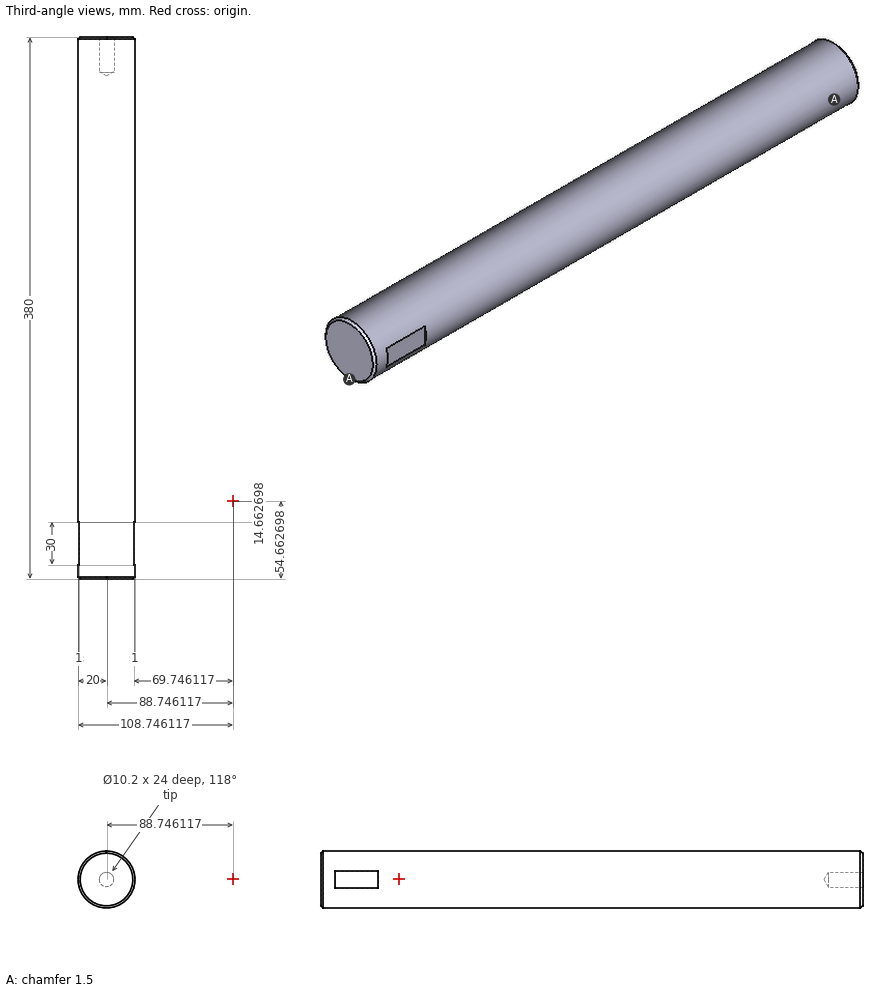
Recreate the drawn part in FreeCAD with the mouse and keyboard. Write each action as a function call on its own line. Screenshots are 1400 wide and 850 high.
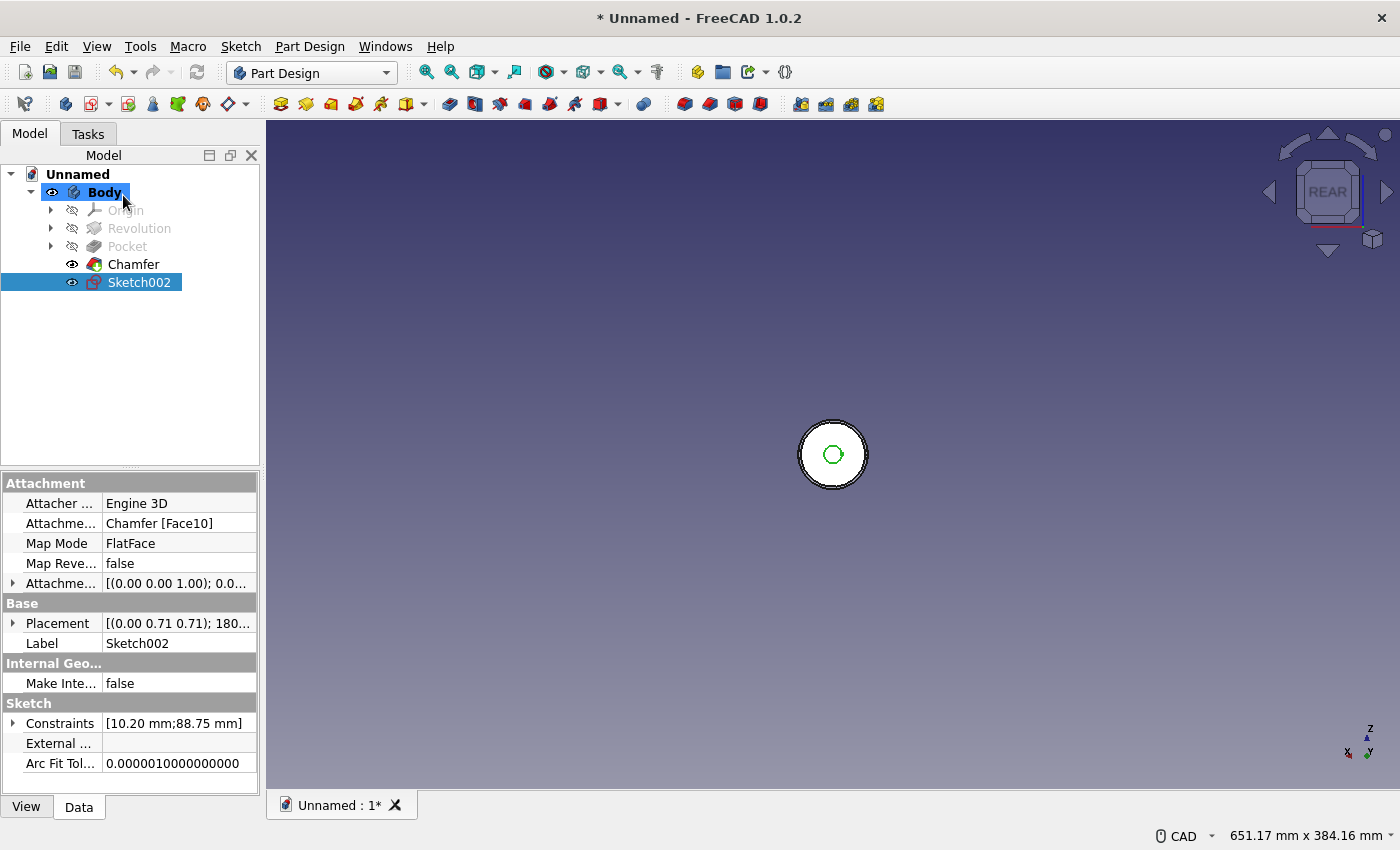
click(475, 104)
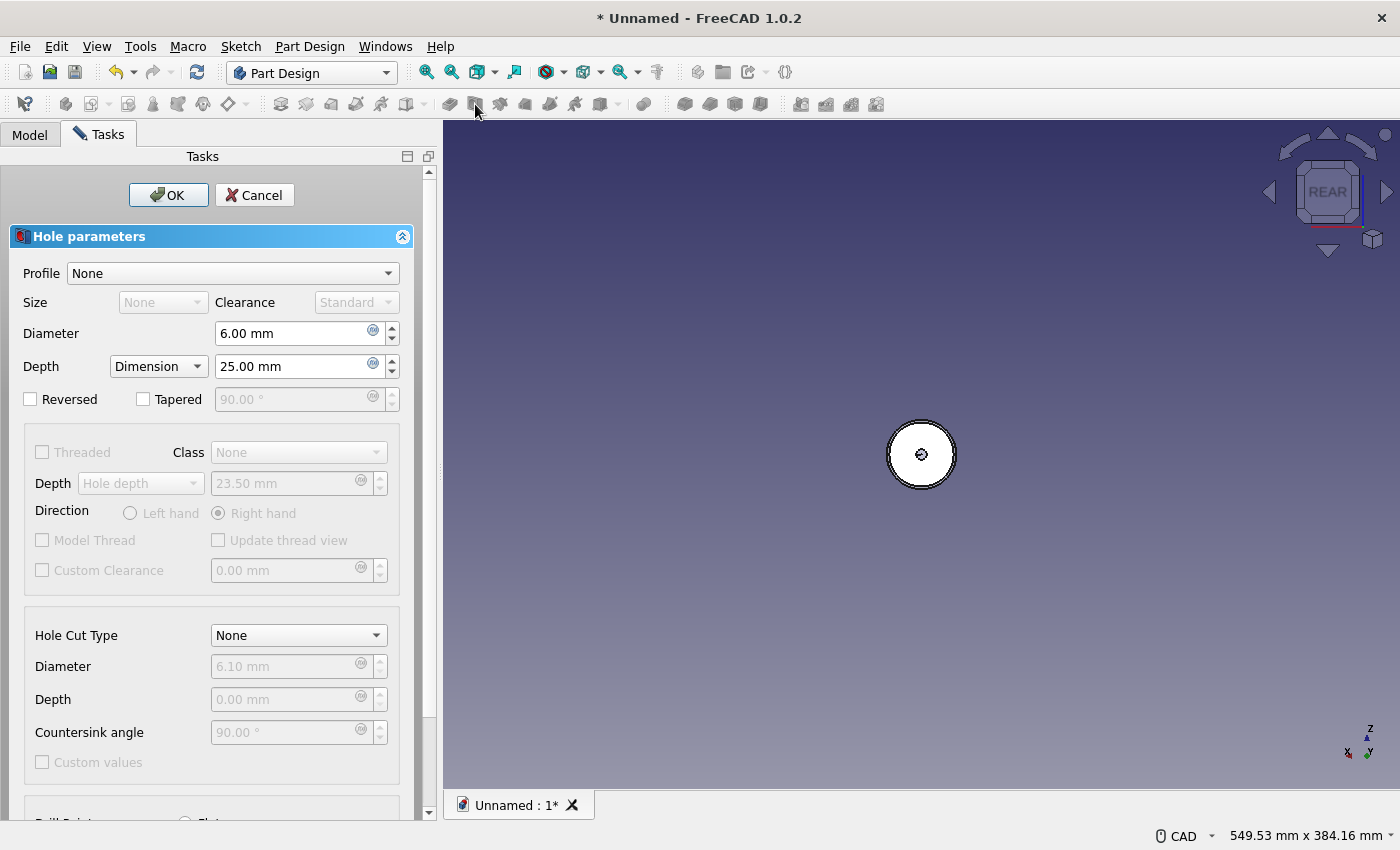
triple_click(300, 334)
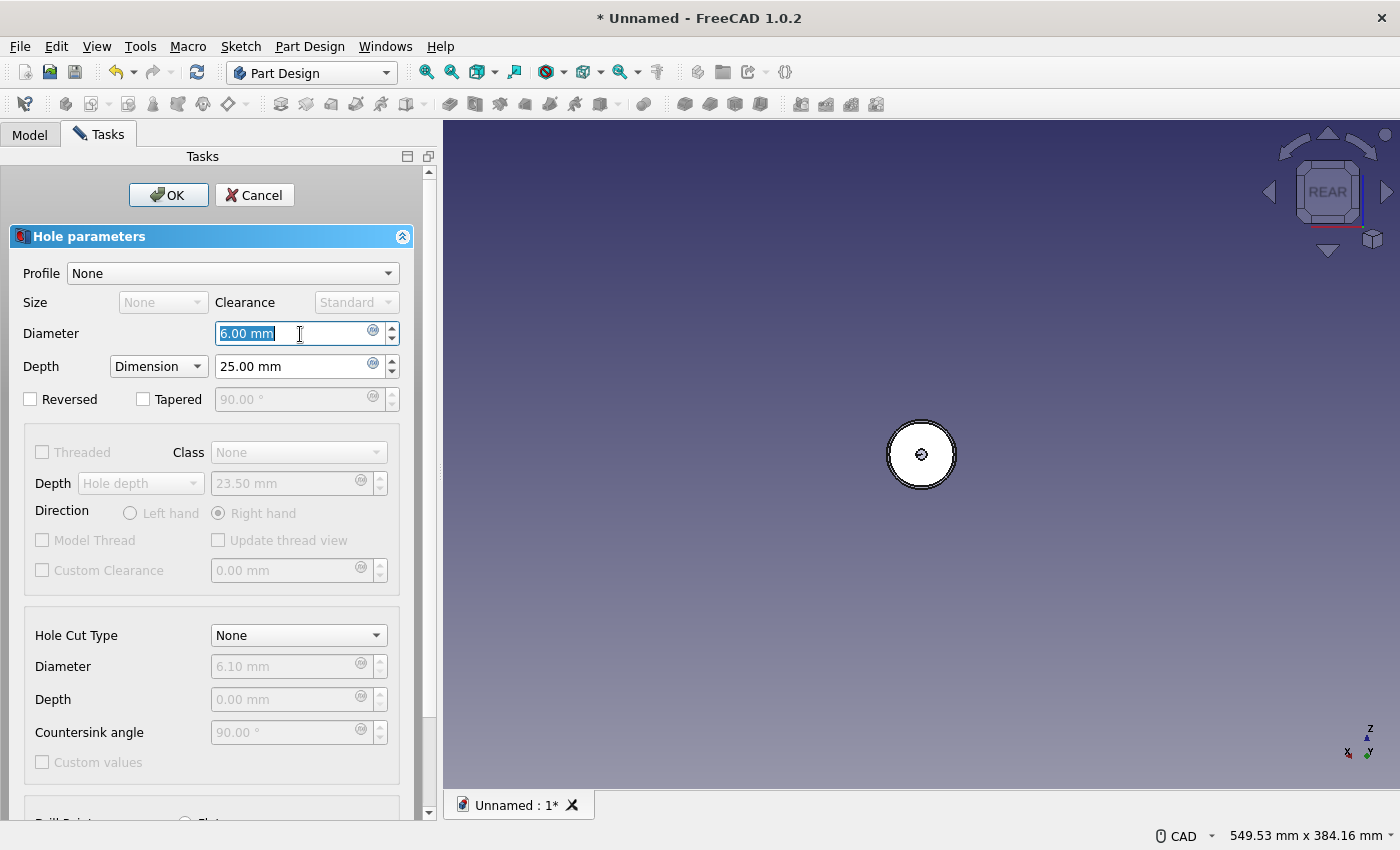
text(10.2)
key(Tab)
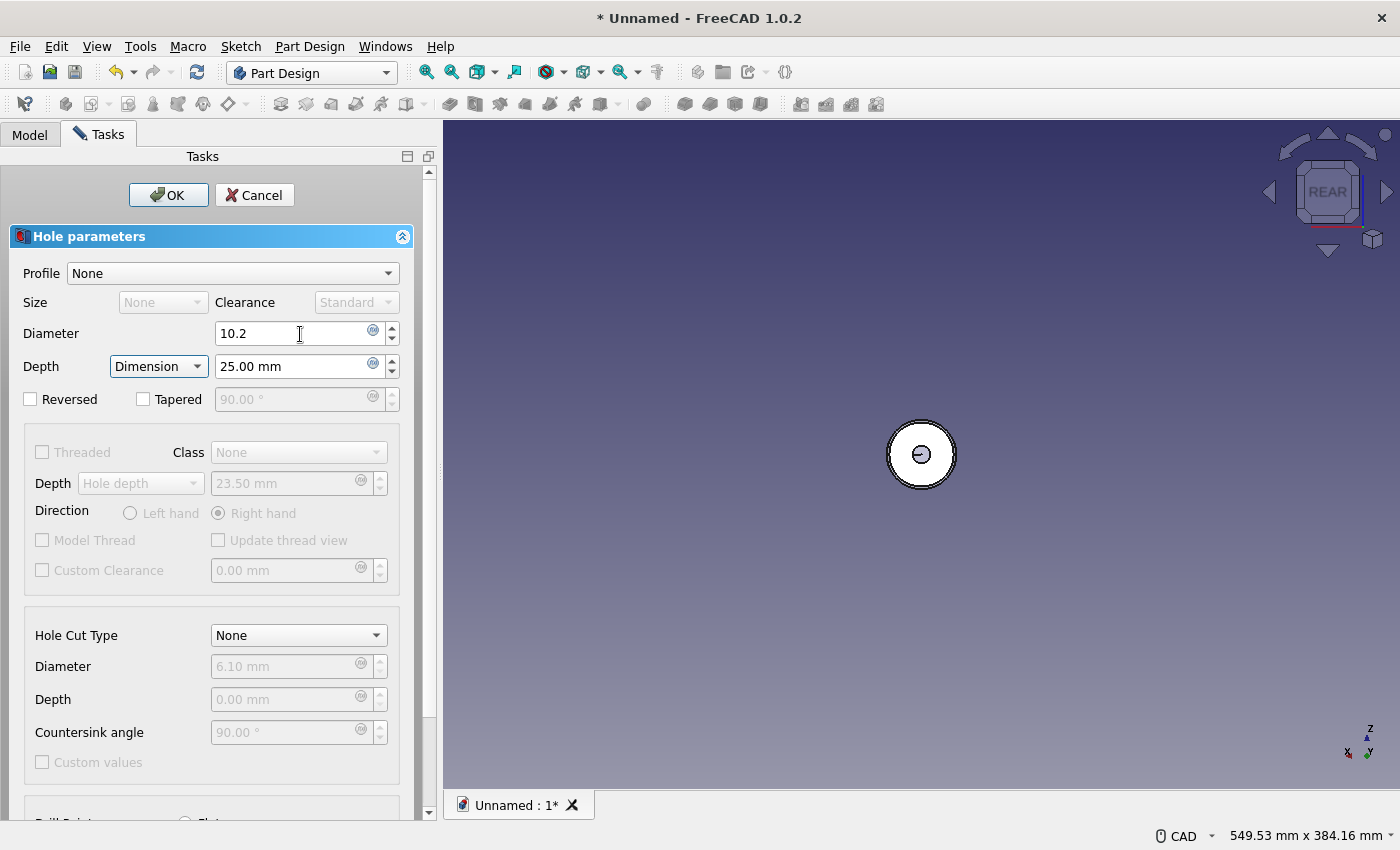
triple_click(300, 366)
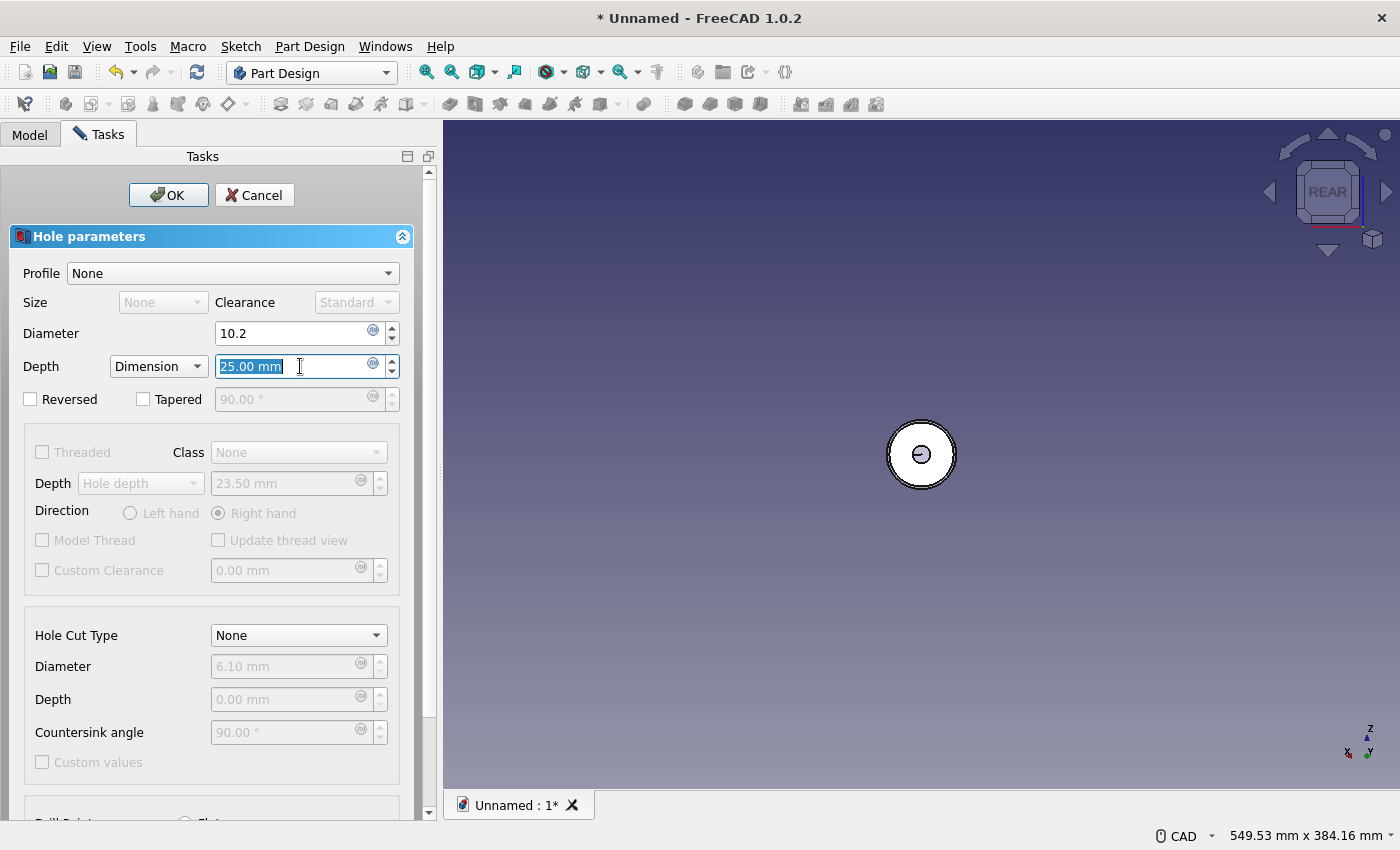
text(24)
key(Tab)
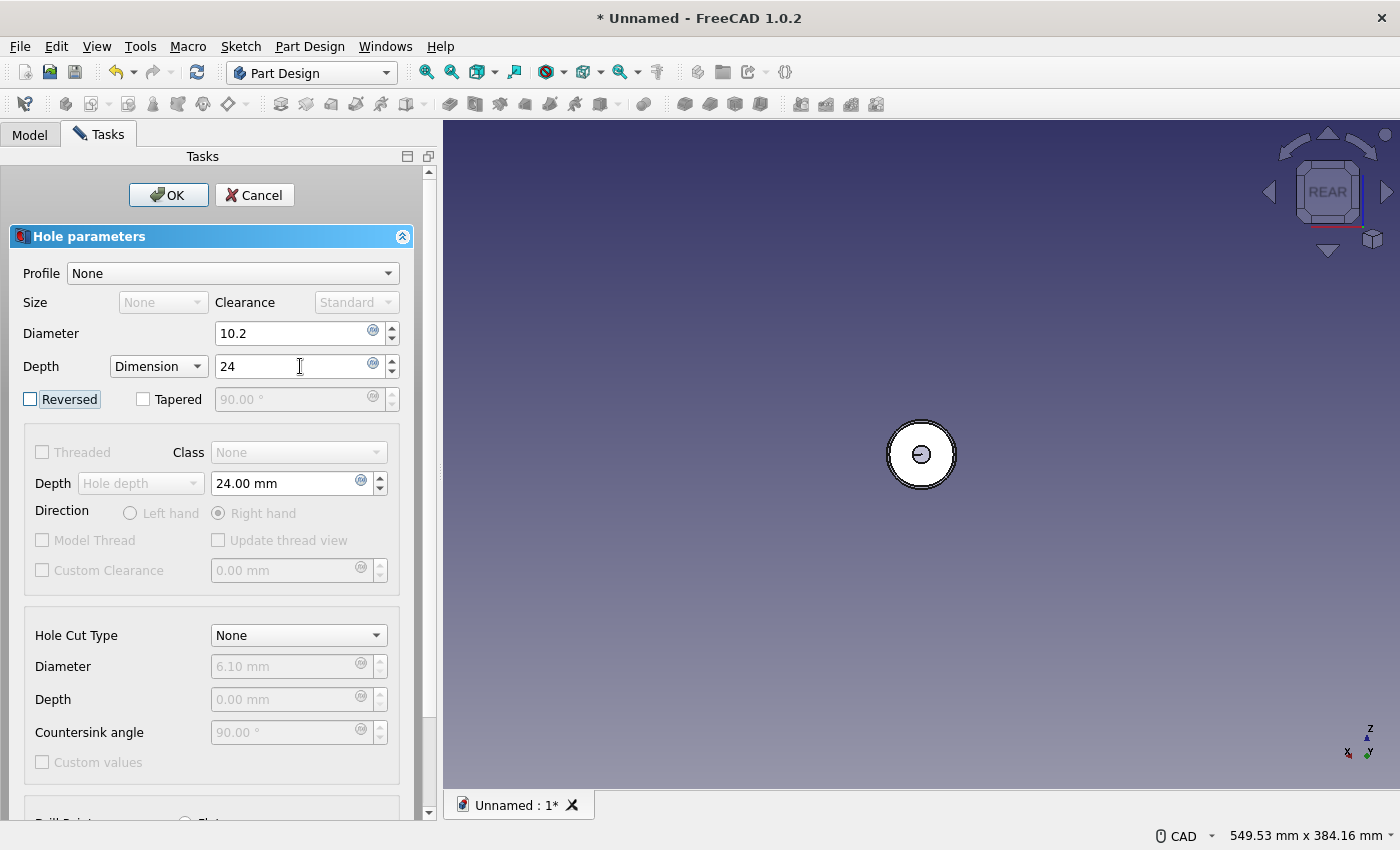
click(169, 195)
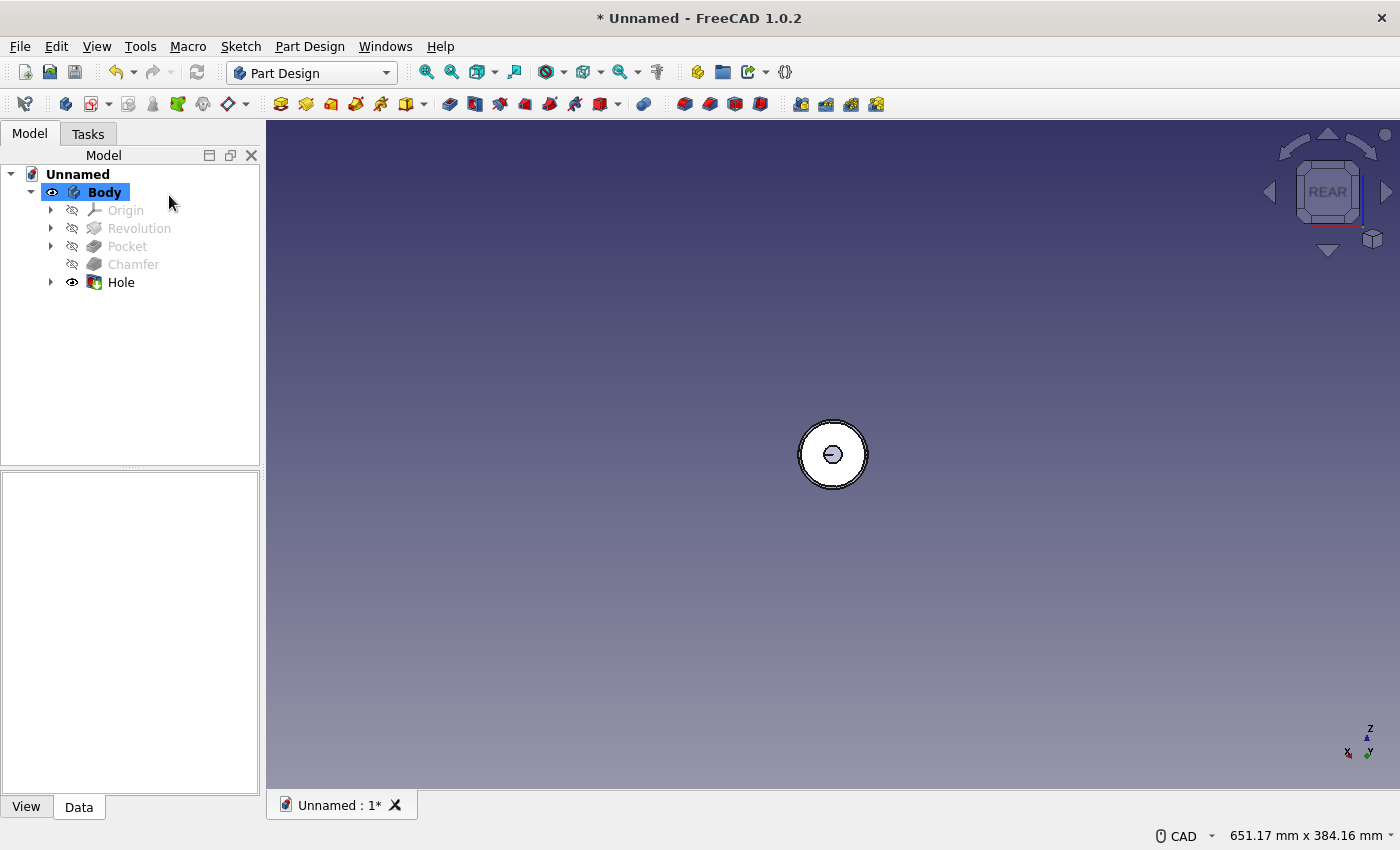
key(0)